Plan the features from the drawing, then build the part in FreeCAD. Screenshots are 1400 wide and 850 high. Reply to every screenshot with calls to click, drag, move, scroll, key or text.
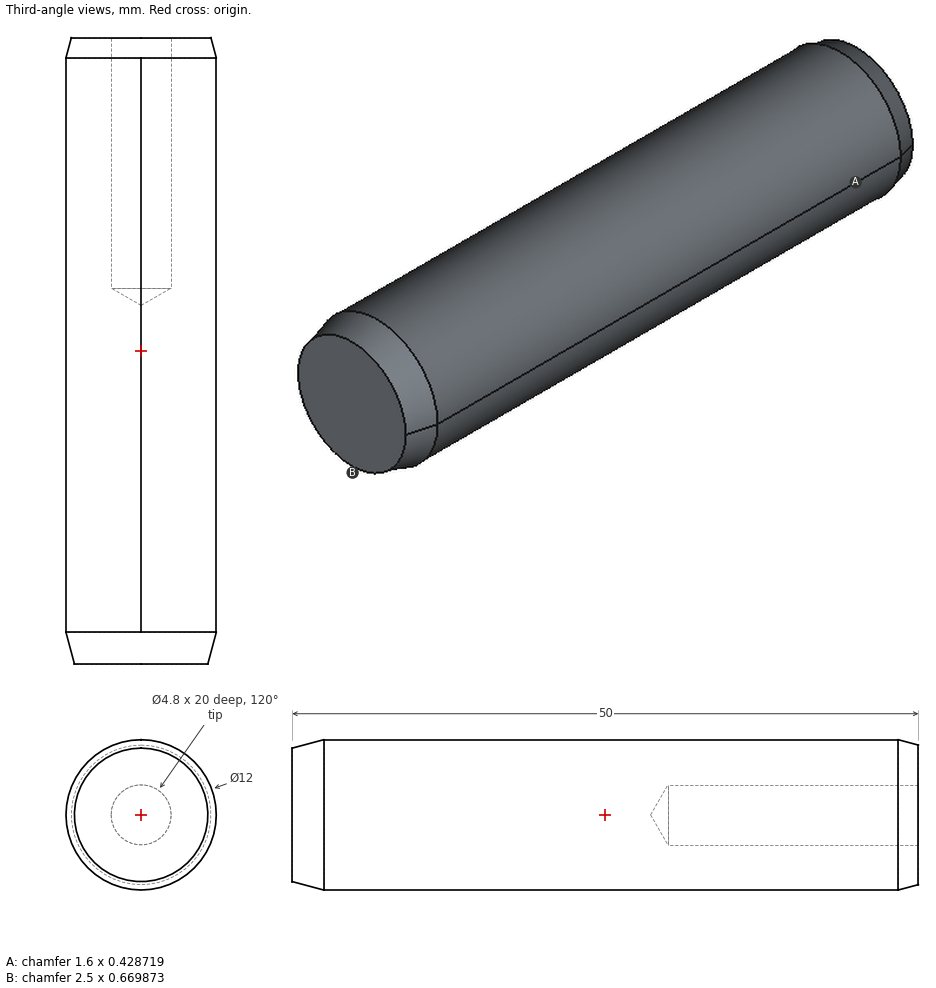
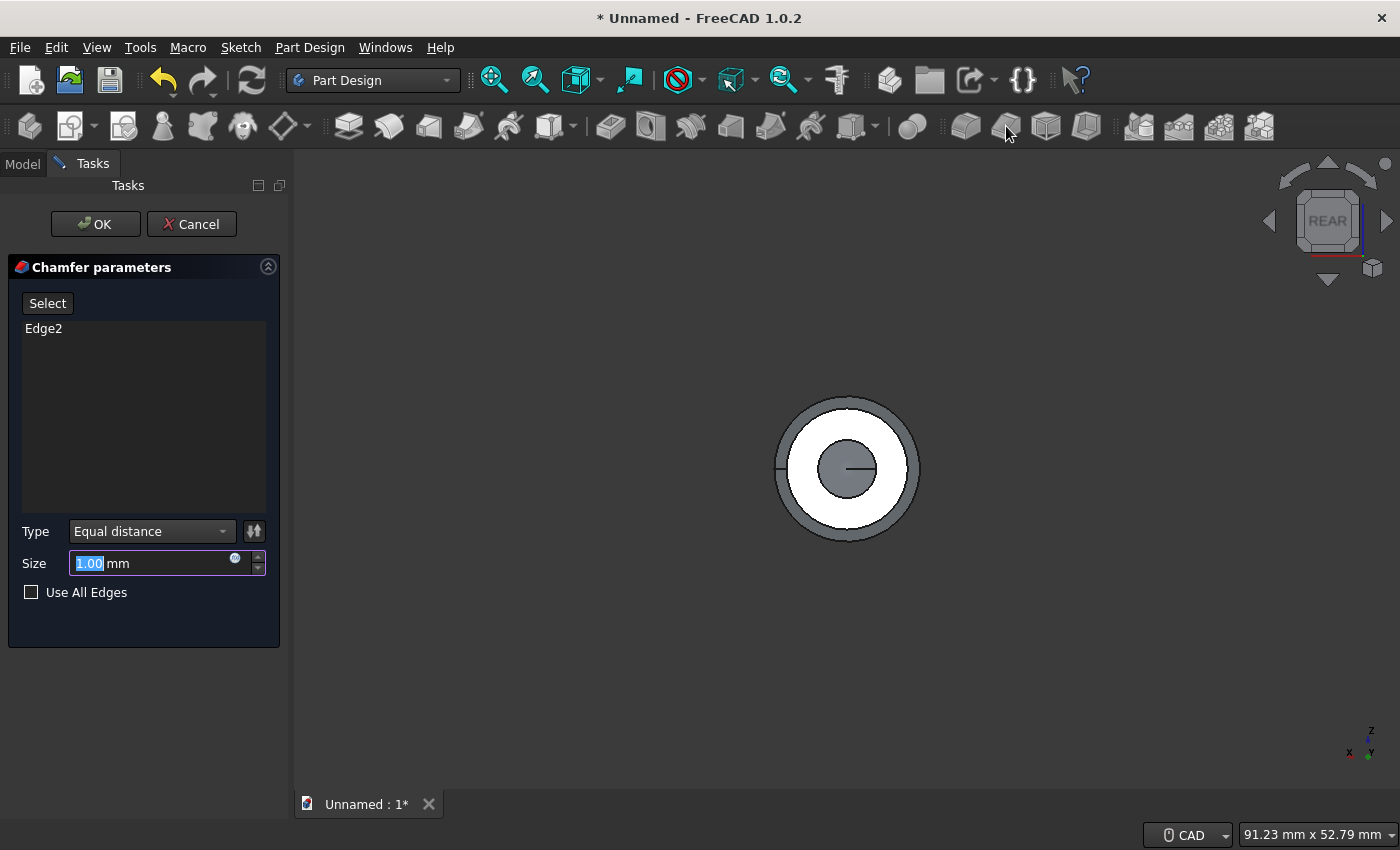
text(1.6)
key(Tab)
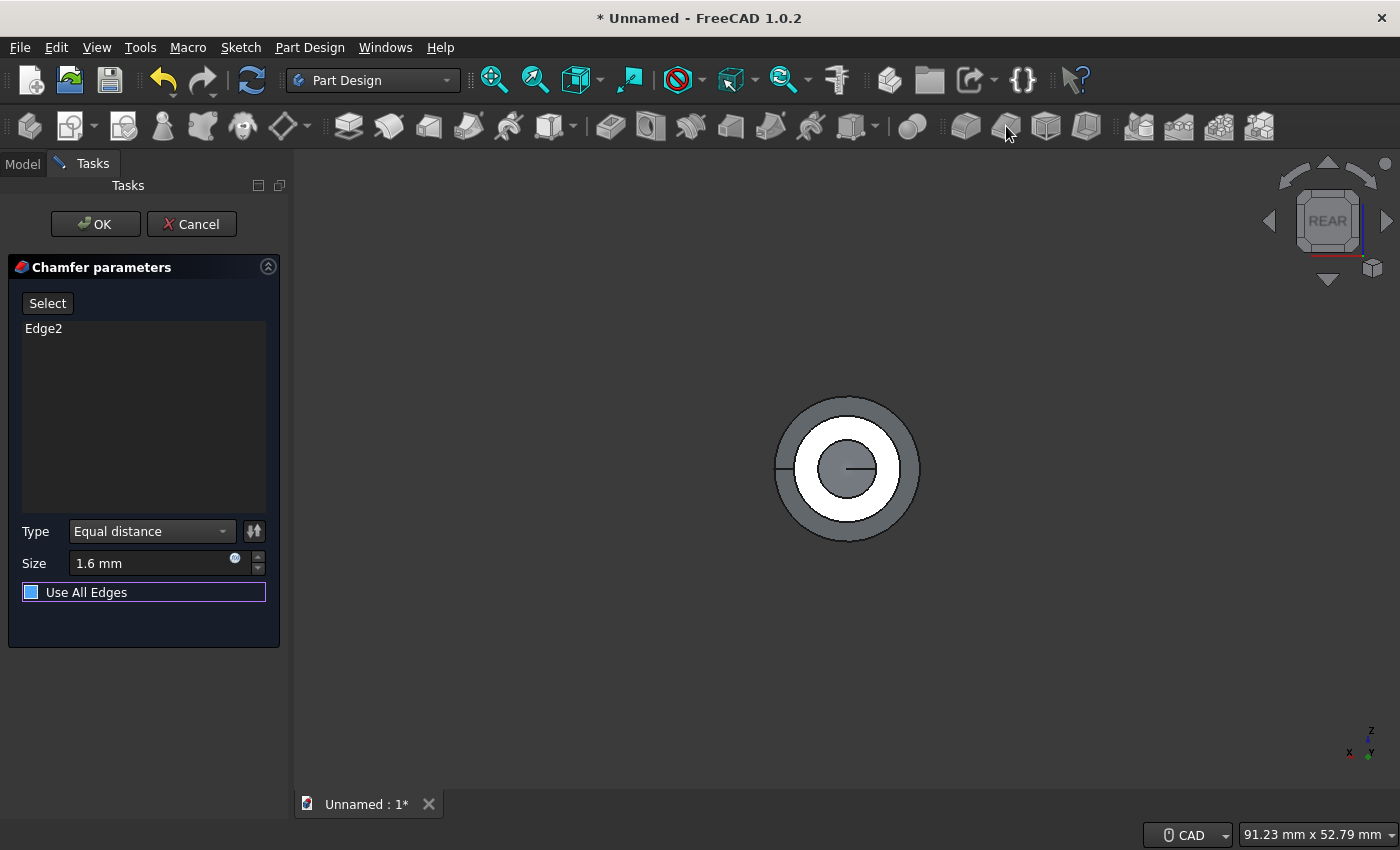
click(153, 532)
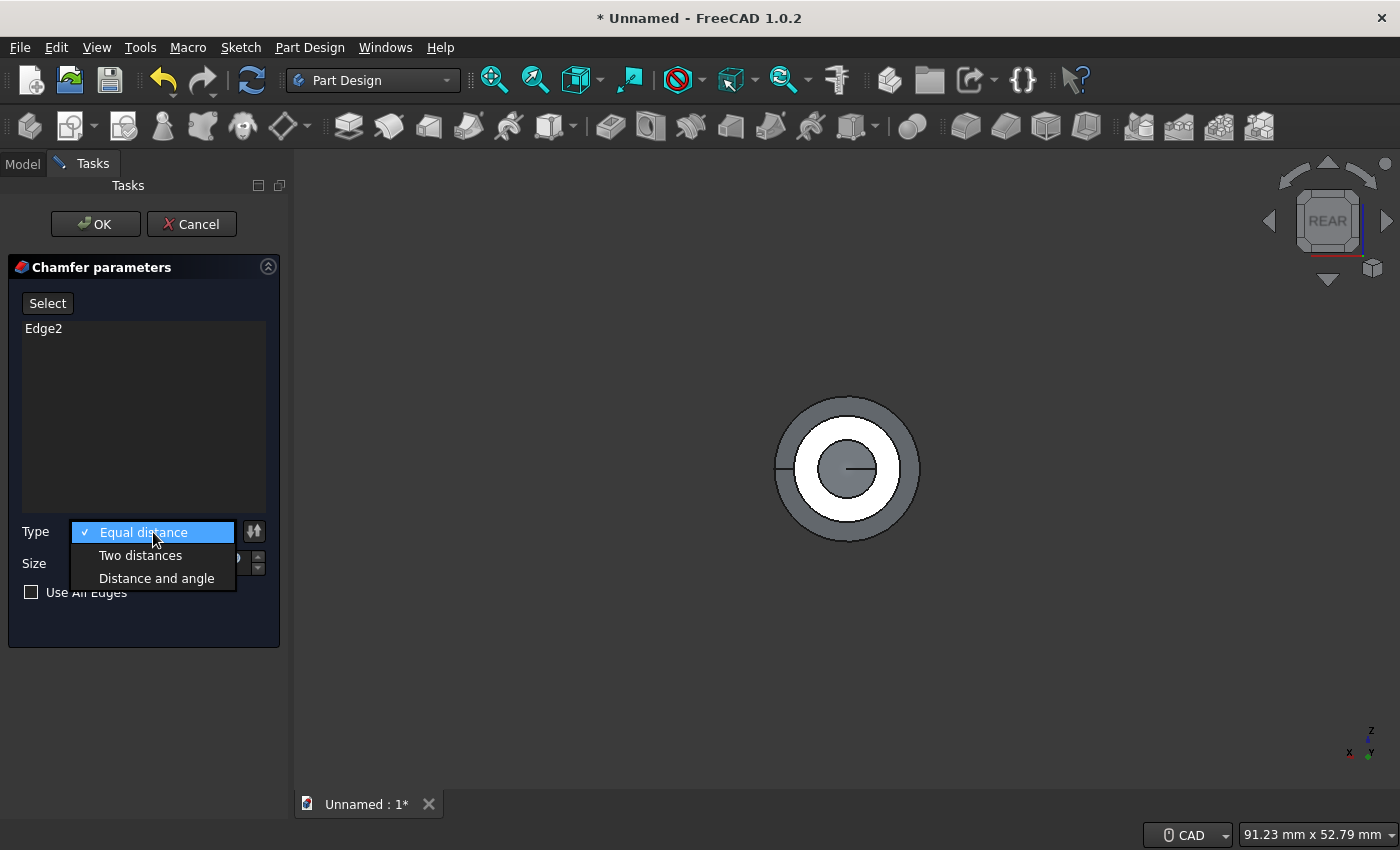
click(152, 556)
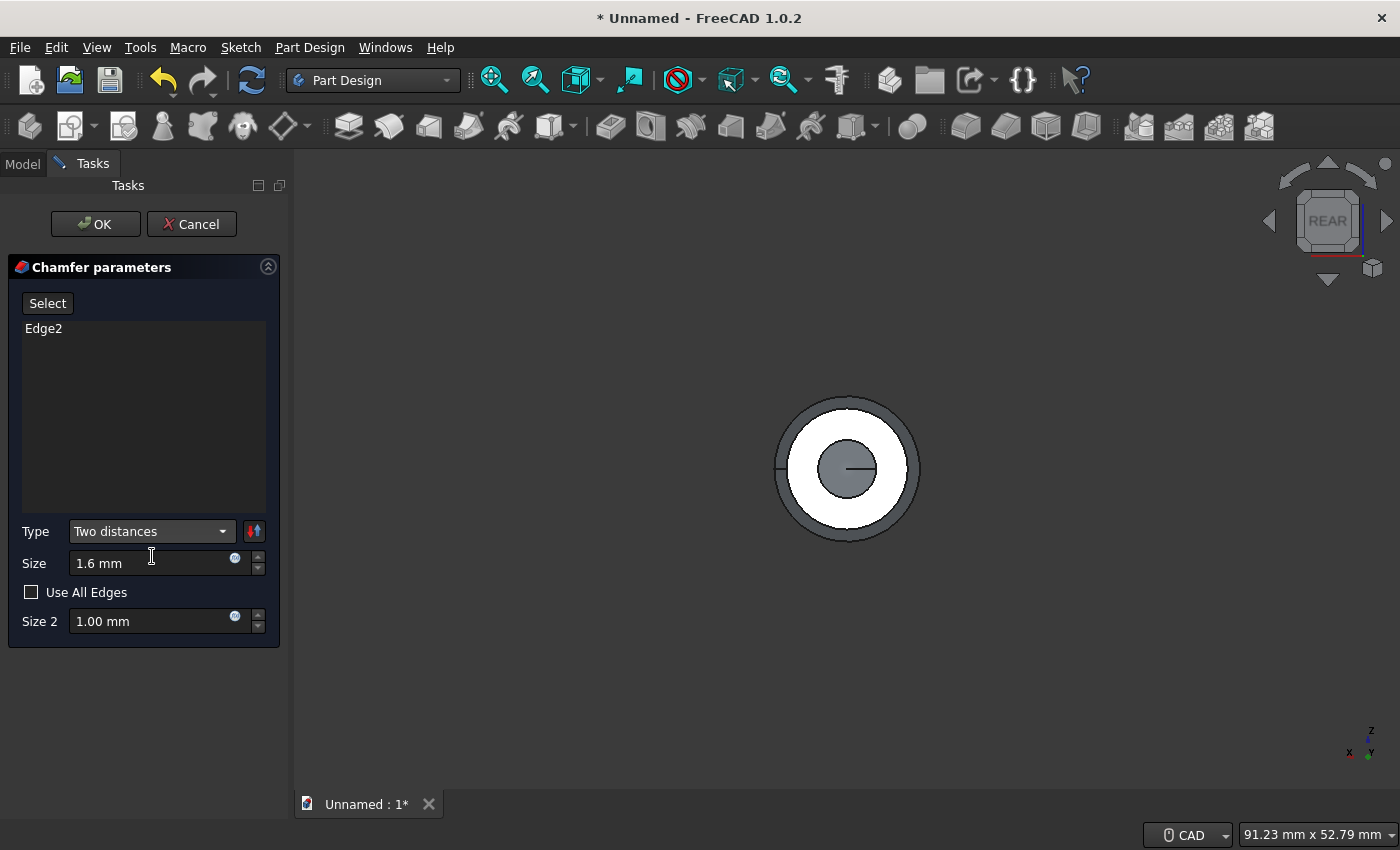
triple_click(160, 621)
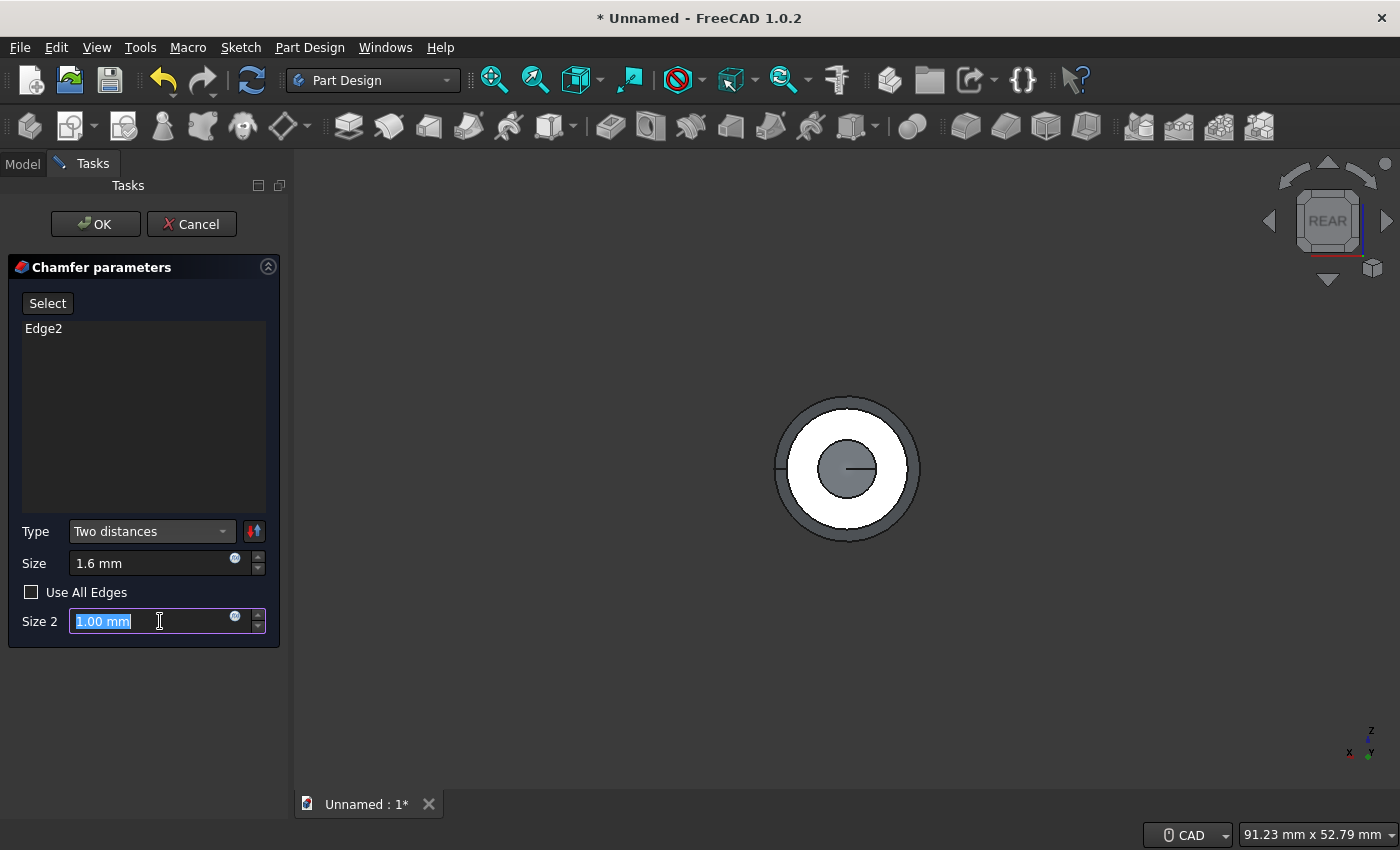
text(0.428719)
key(Tab)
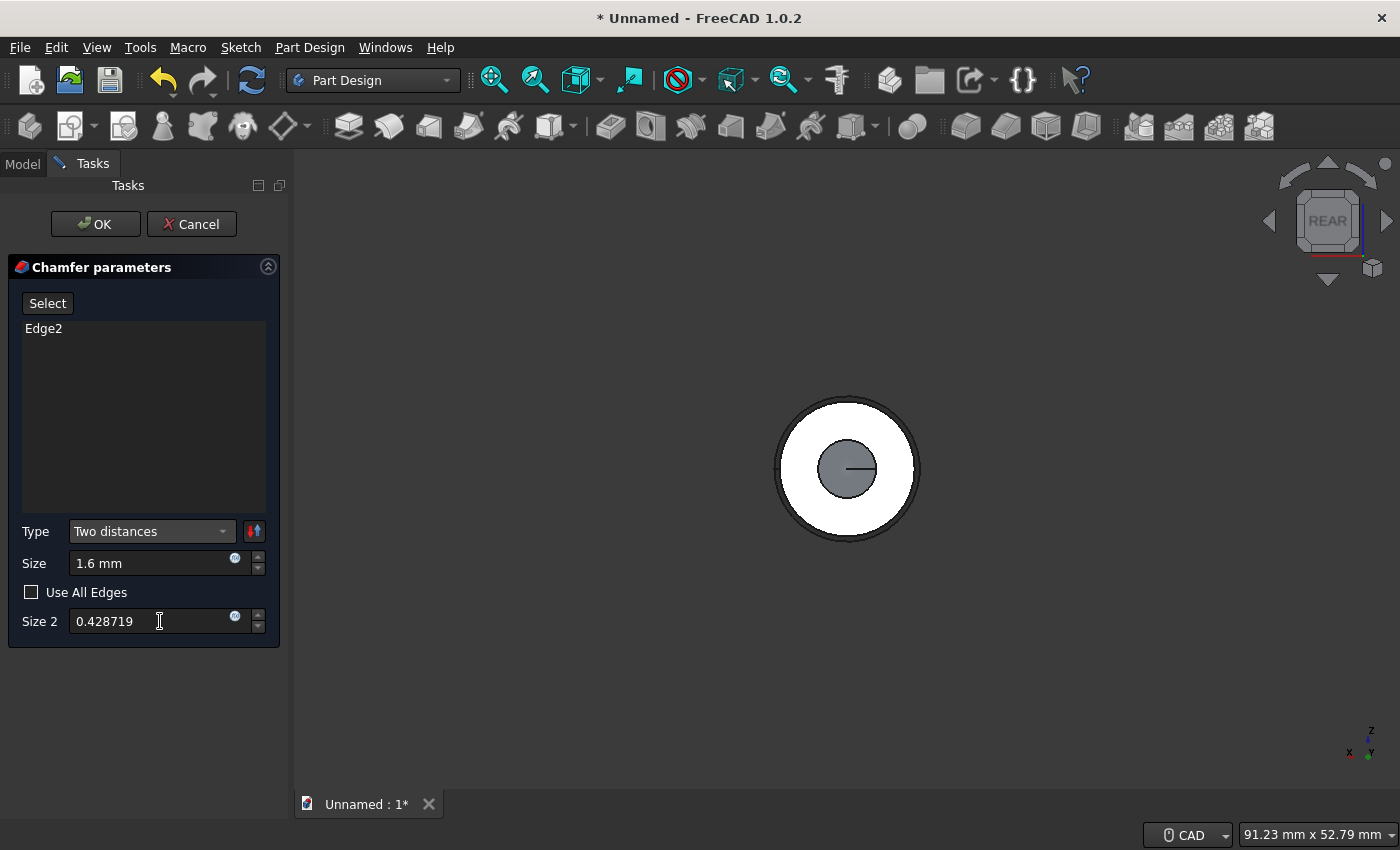
click(96, 224)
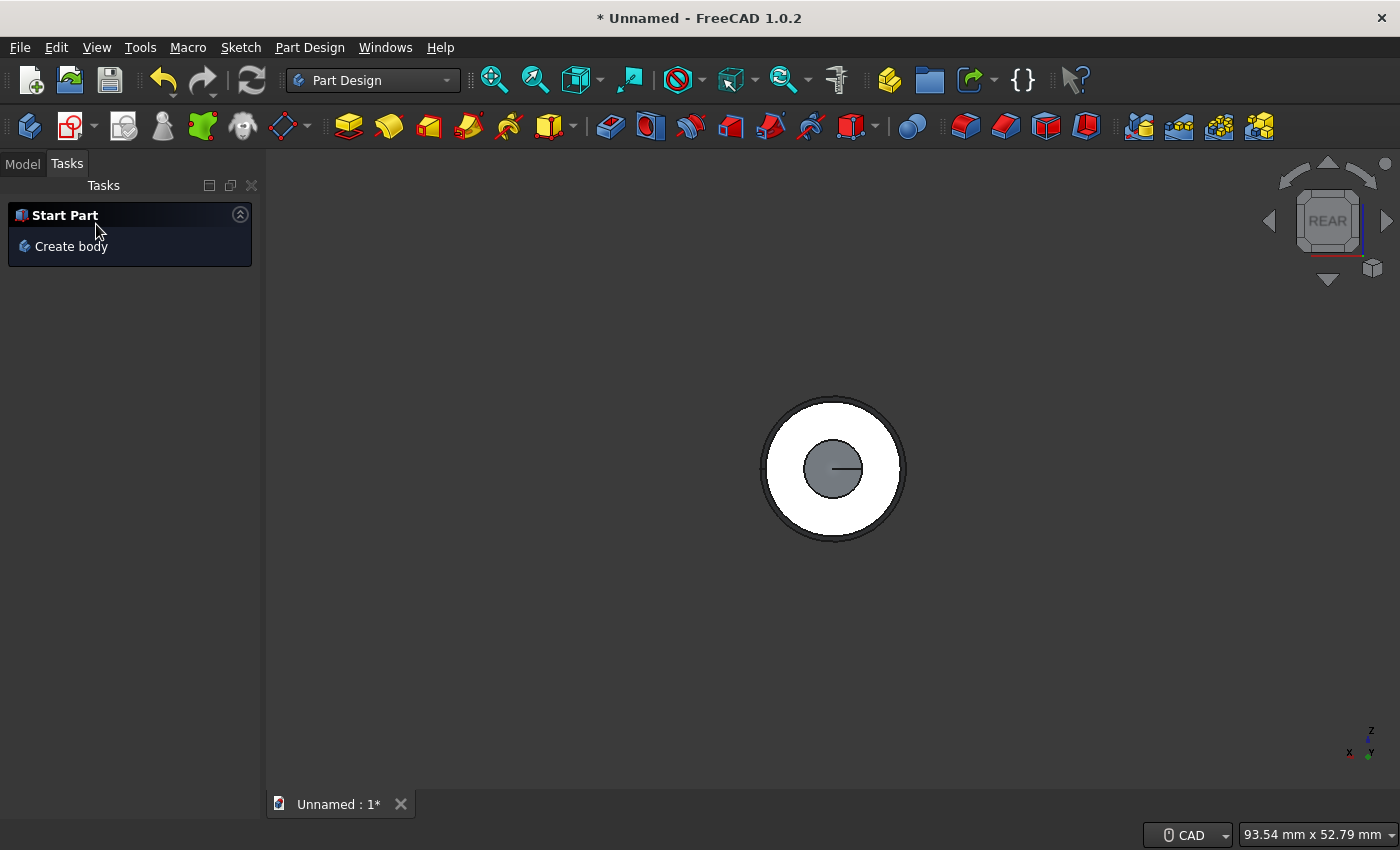
click(496, 80)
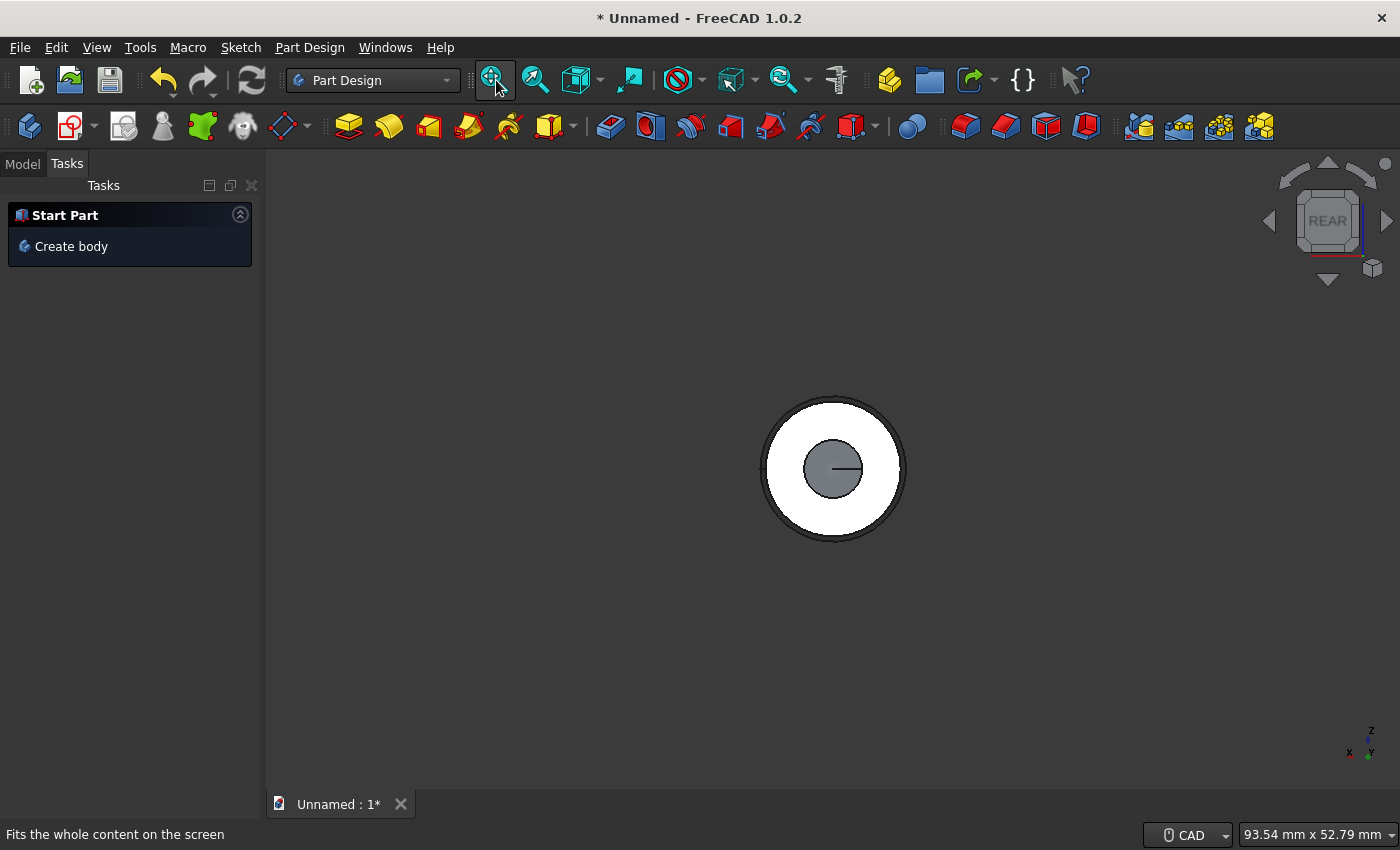
key(0)